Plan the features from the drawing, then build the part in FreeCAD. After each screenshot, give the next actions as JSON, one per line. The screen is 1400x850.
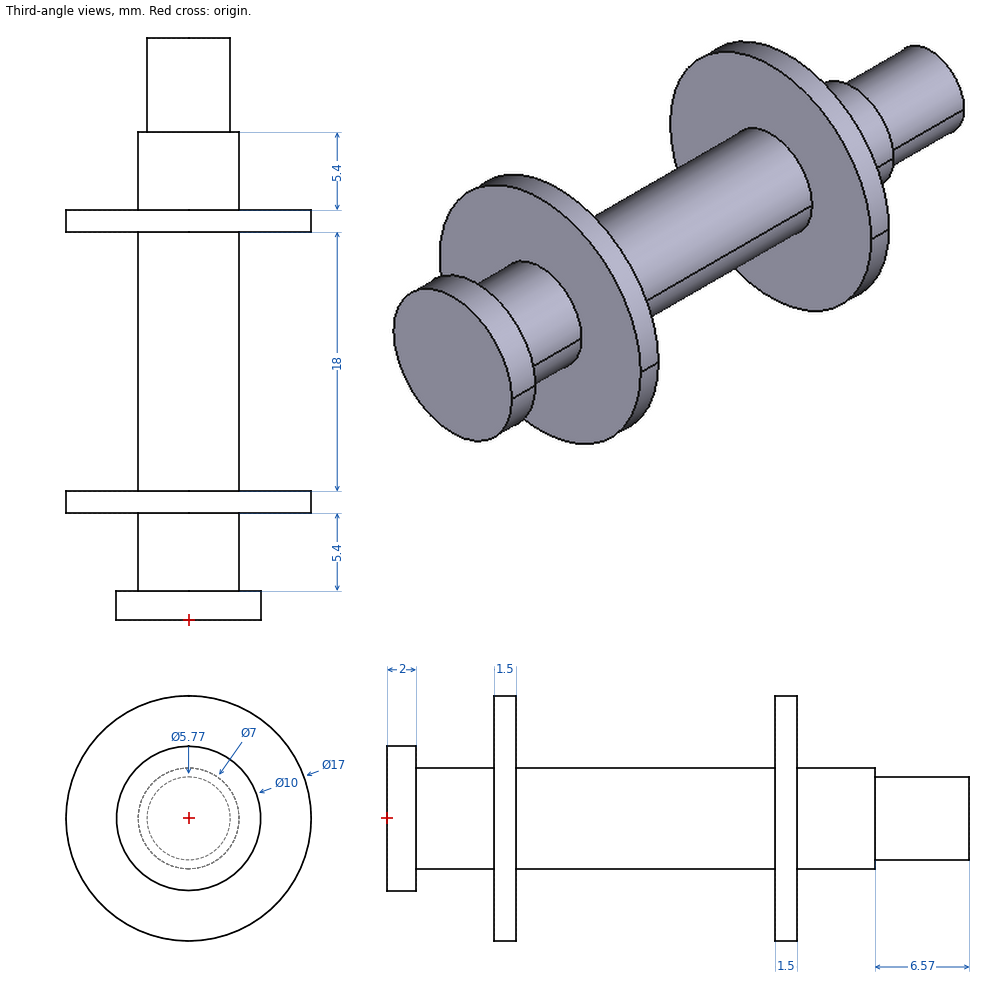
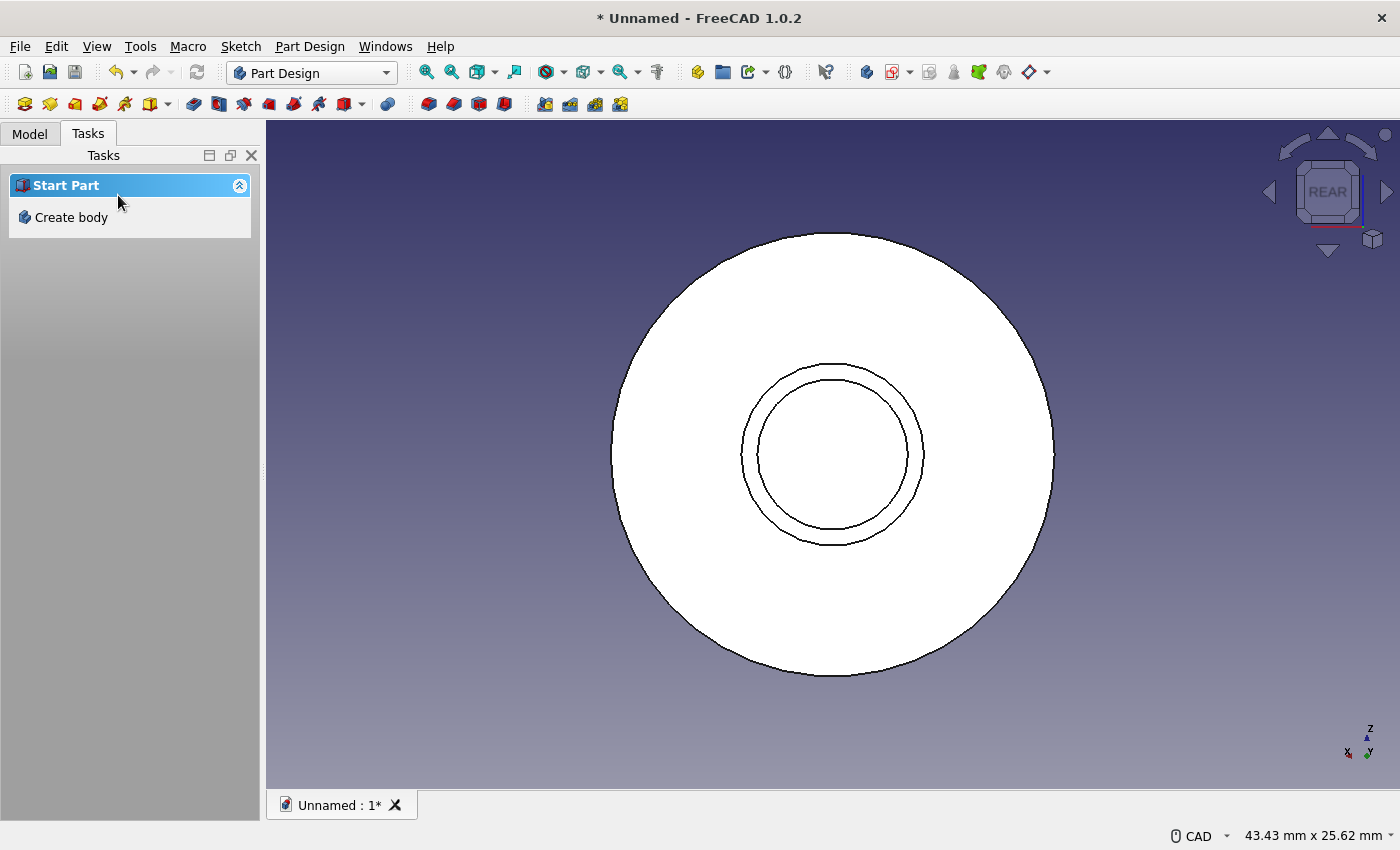
{"action": "key", "text": "0"}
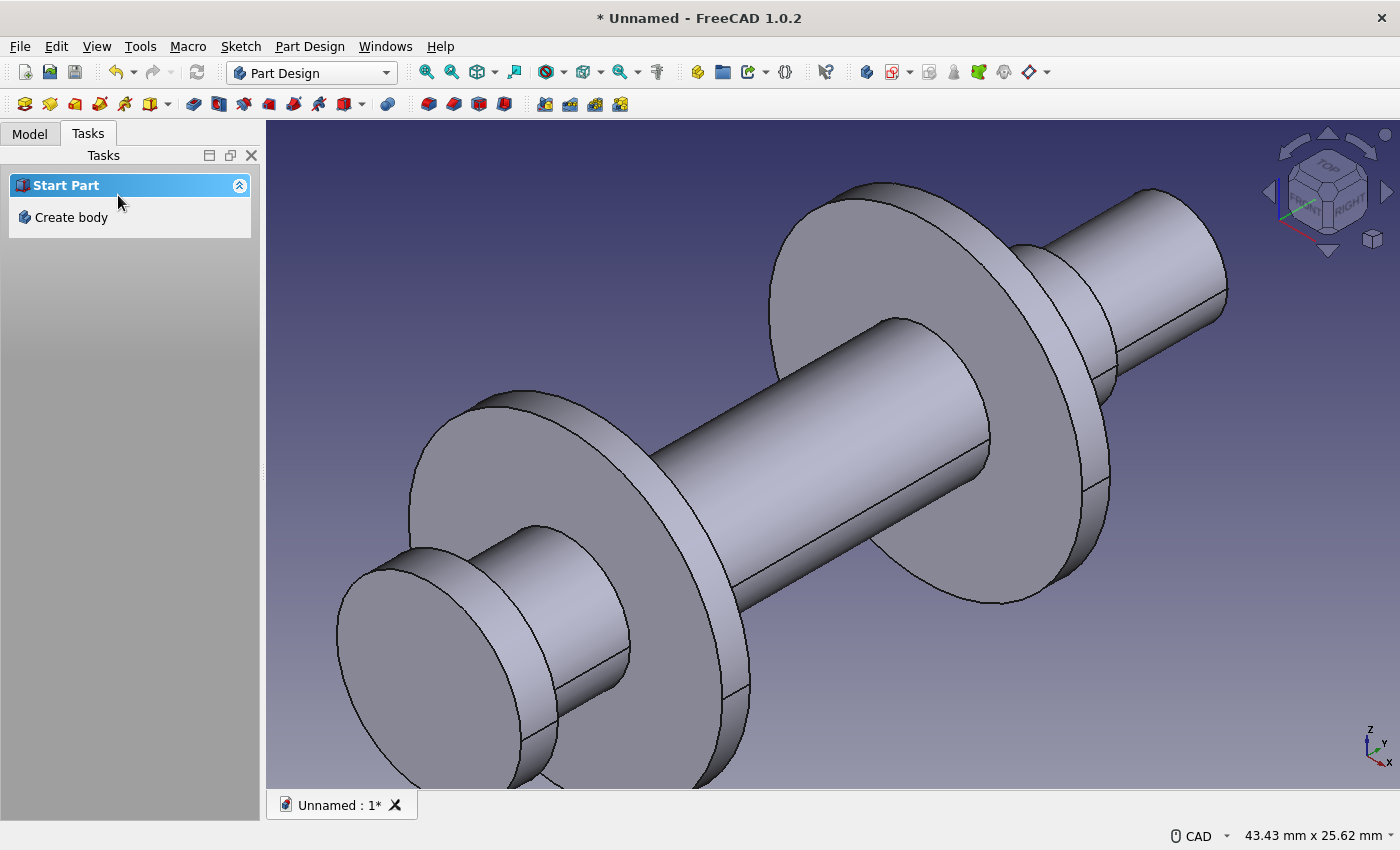
{"action": "left_click", "coordinate": [427, 72]}